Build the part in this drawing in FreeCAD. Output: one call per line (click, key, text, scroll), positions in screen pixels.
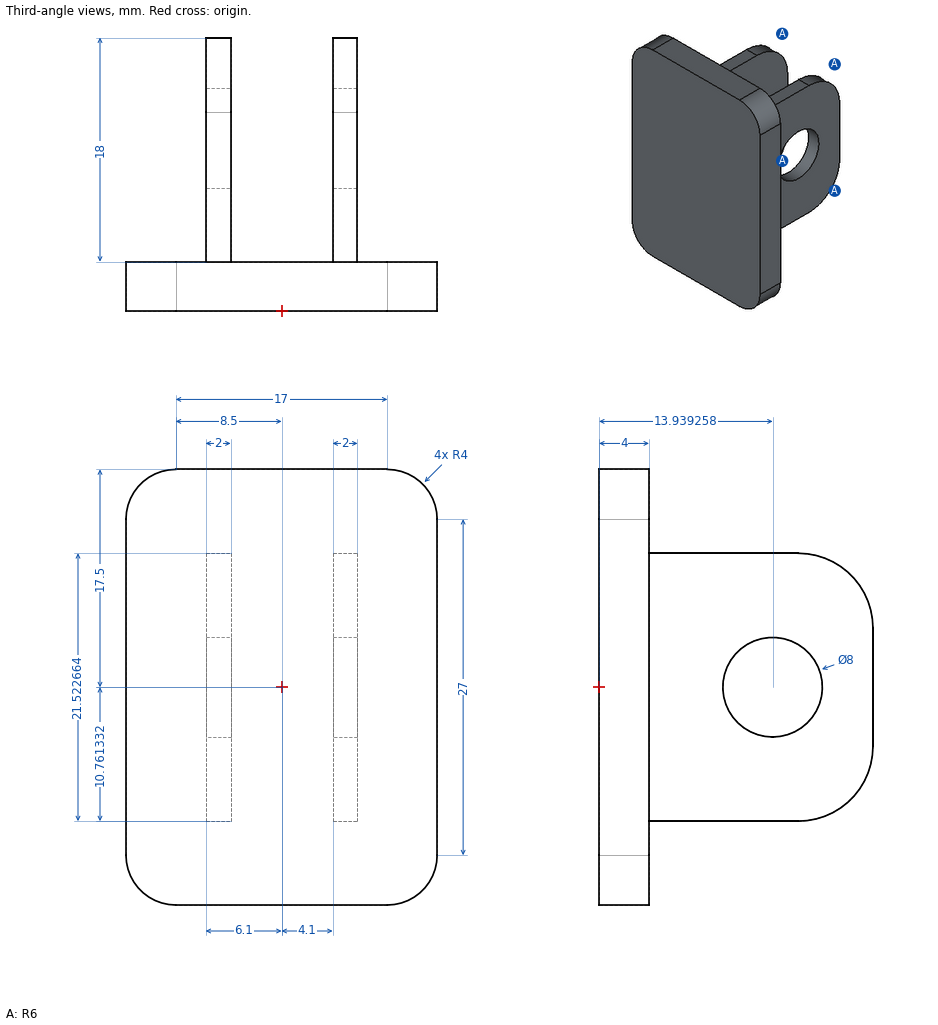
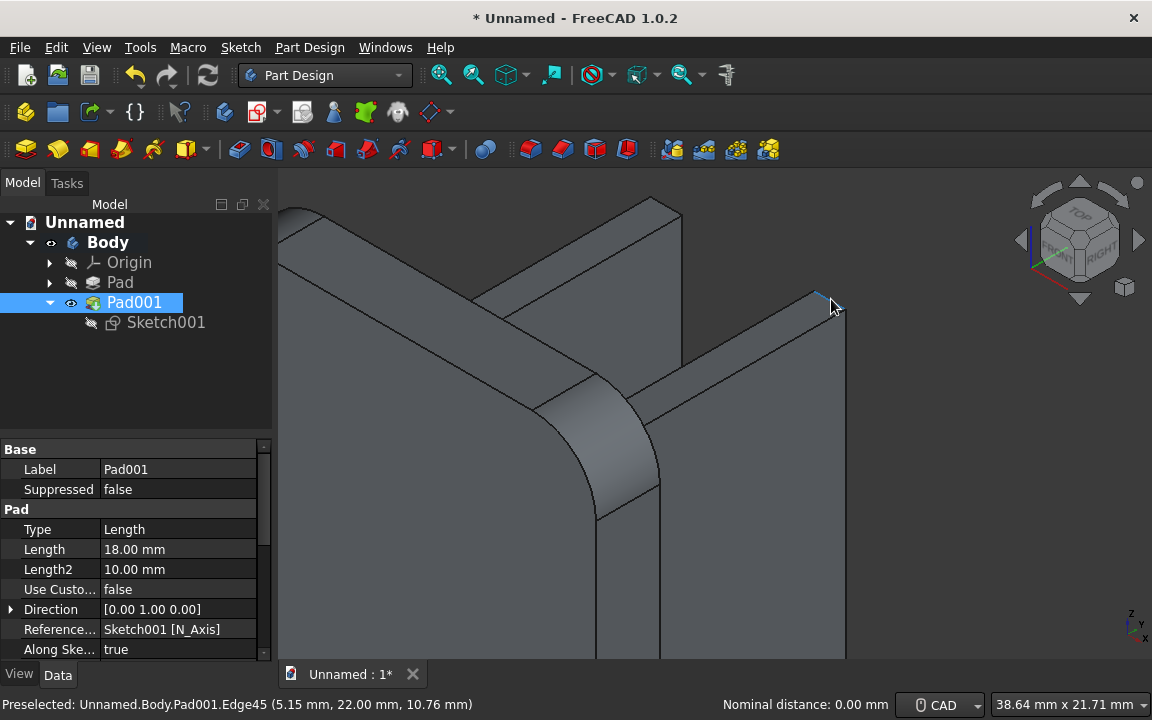
click(442, 76)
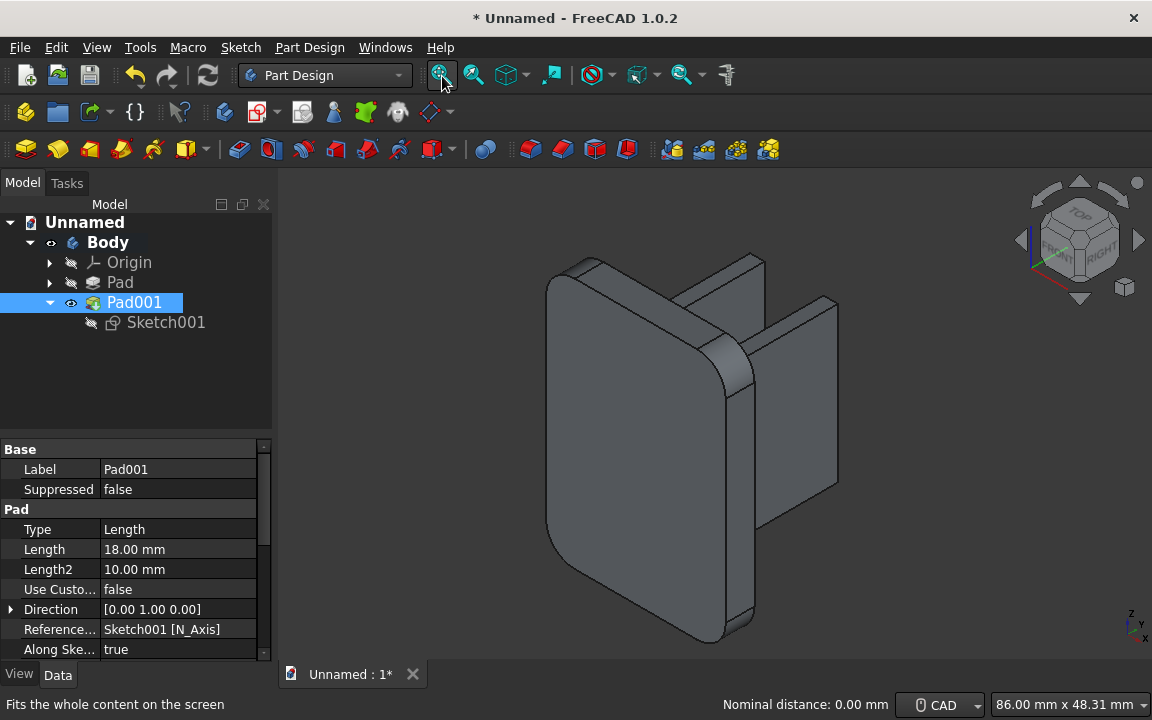
key(2)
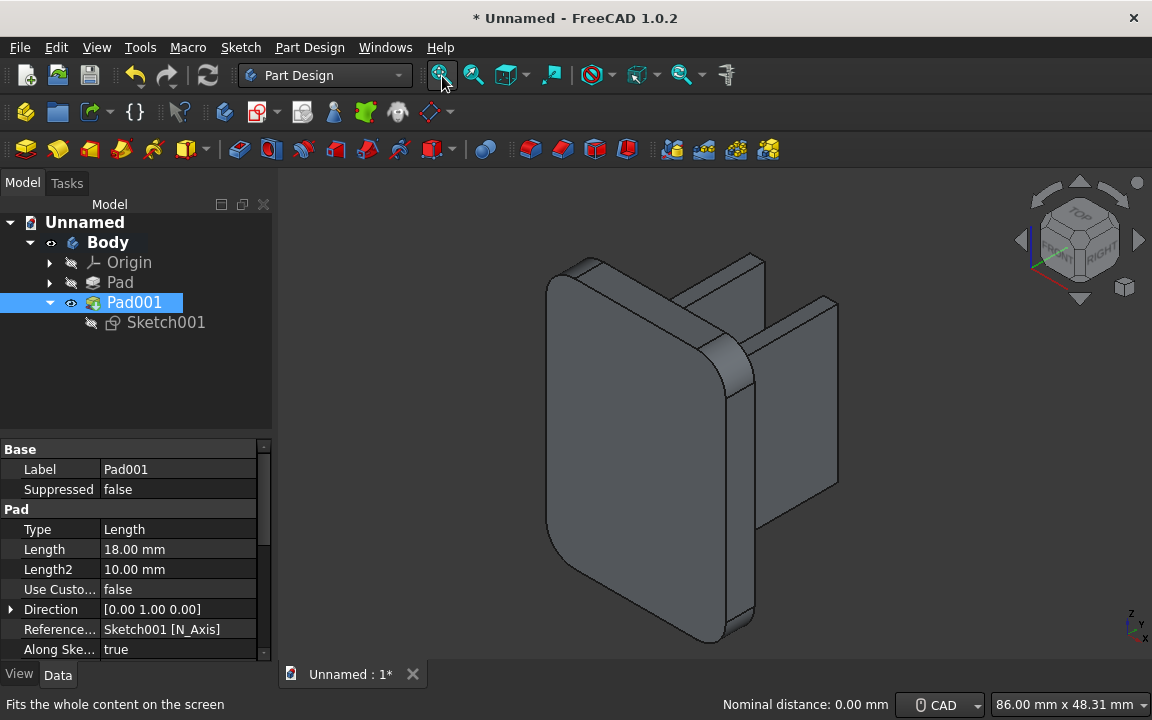
click(767, 301, ctrl)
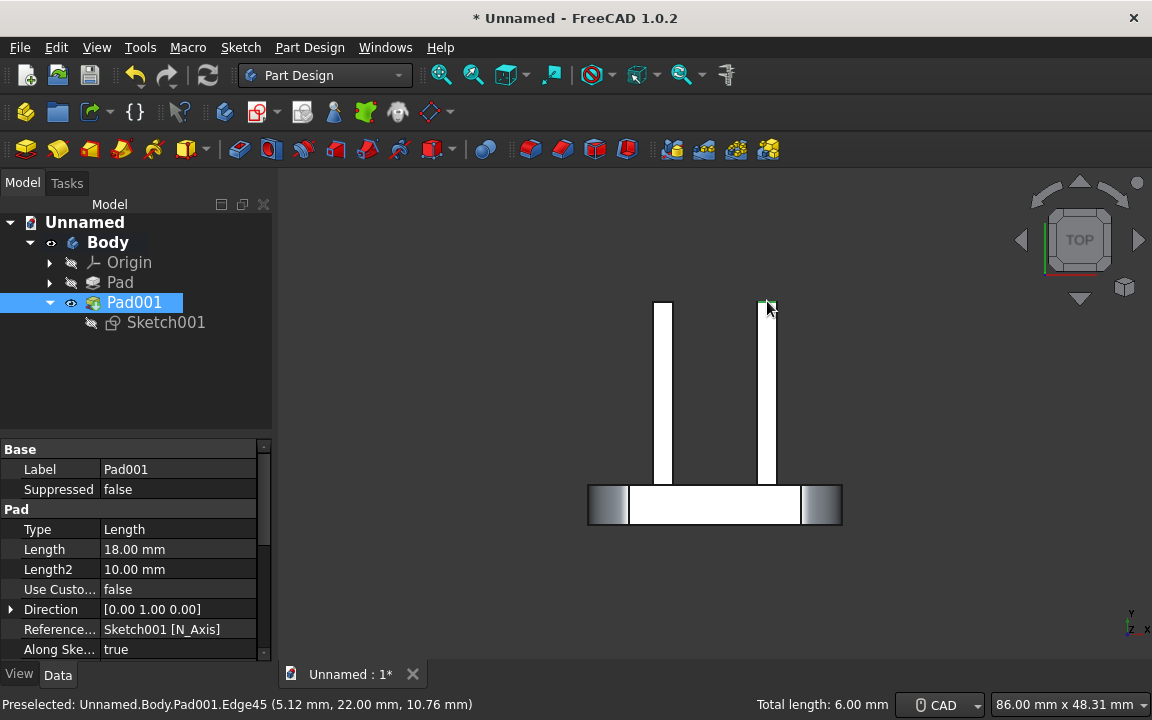
click(663, 301, ctrl)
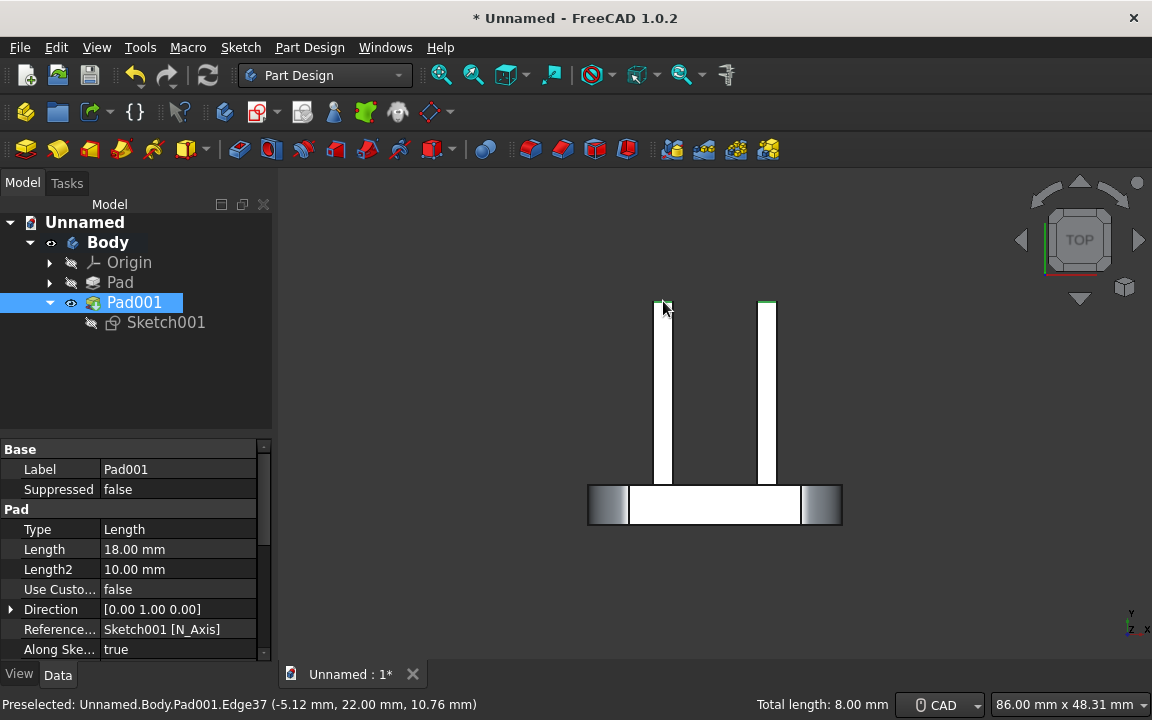
click(532, 150)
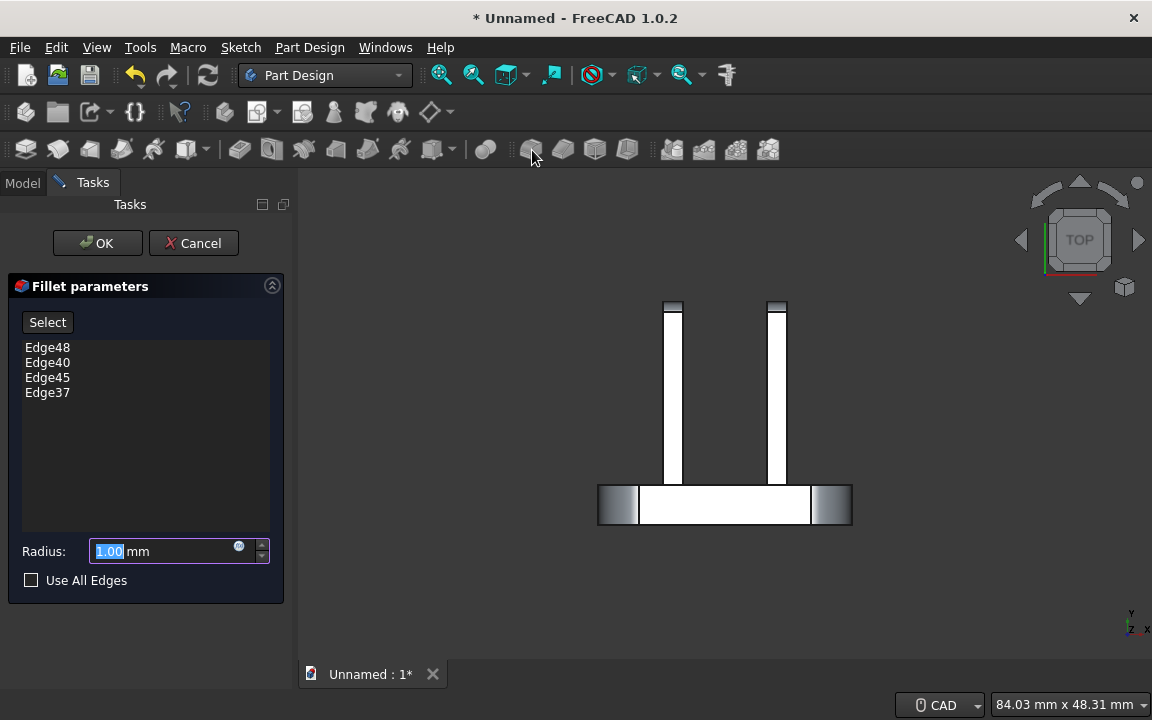
text(6)
key(Tab)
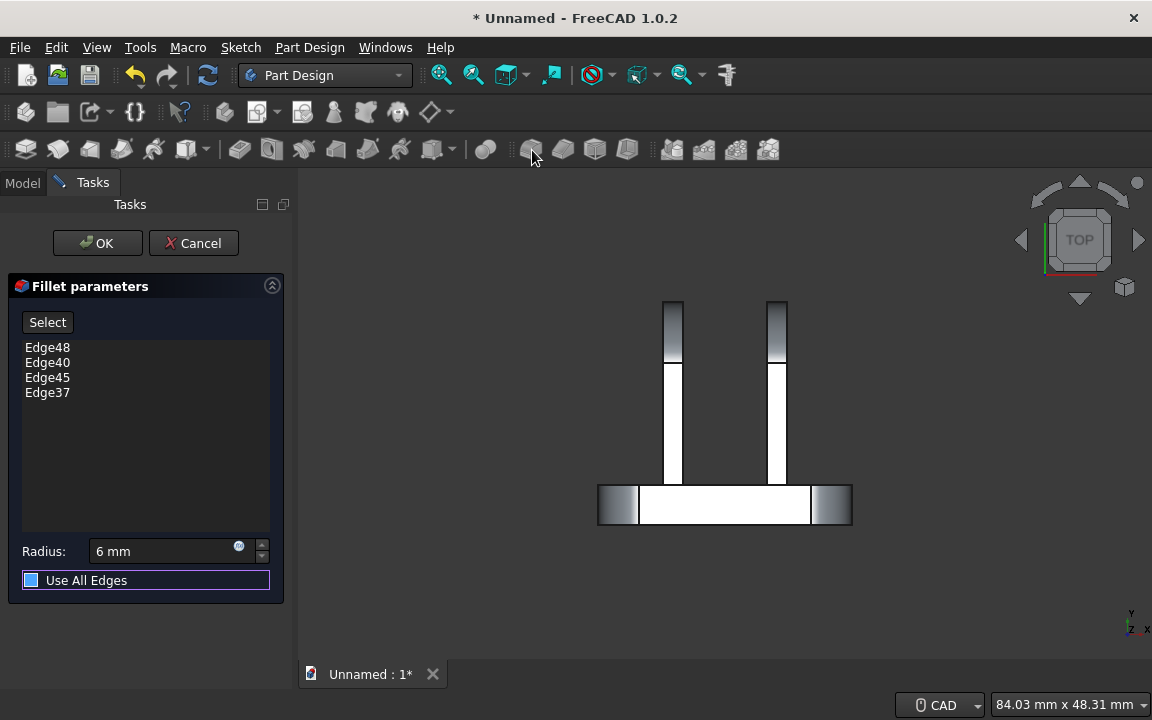
click(98, 243)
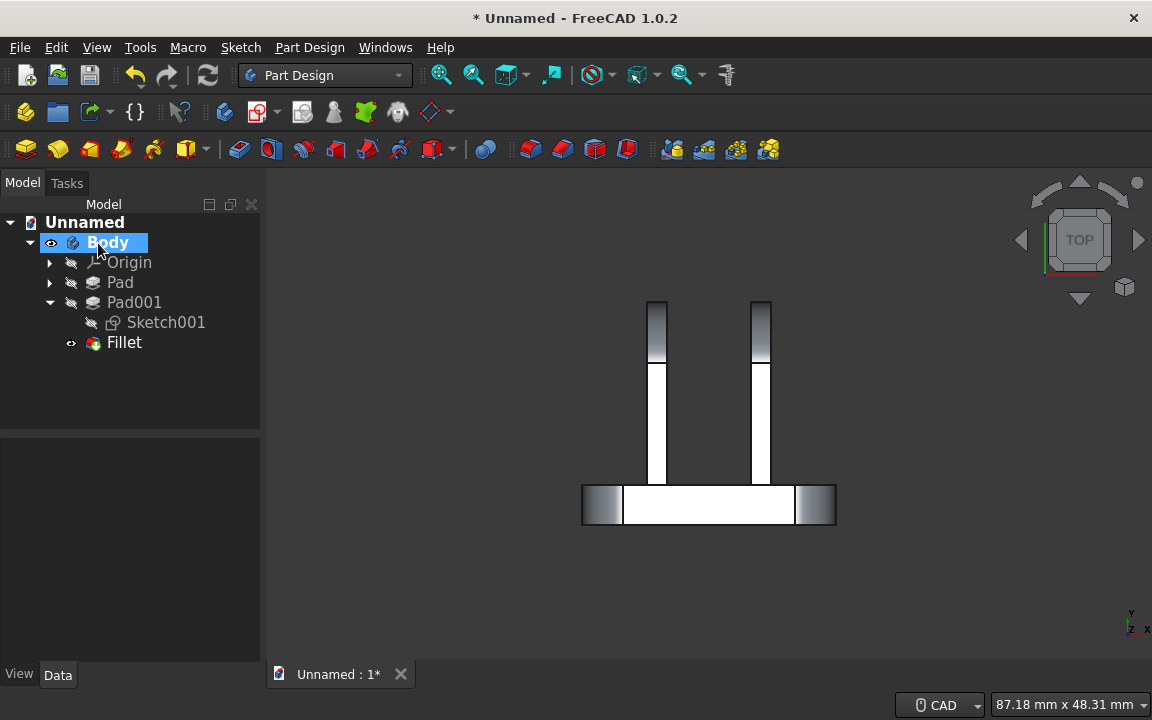
key(0)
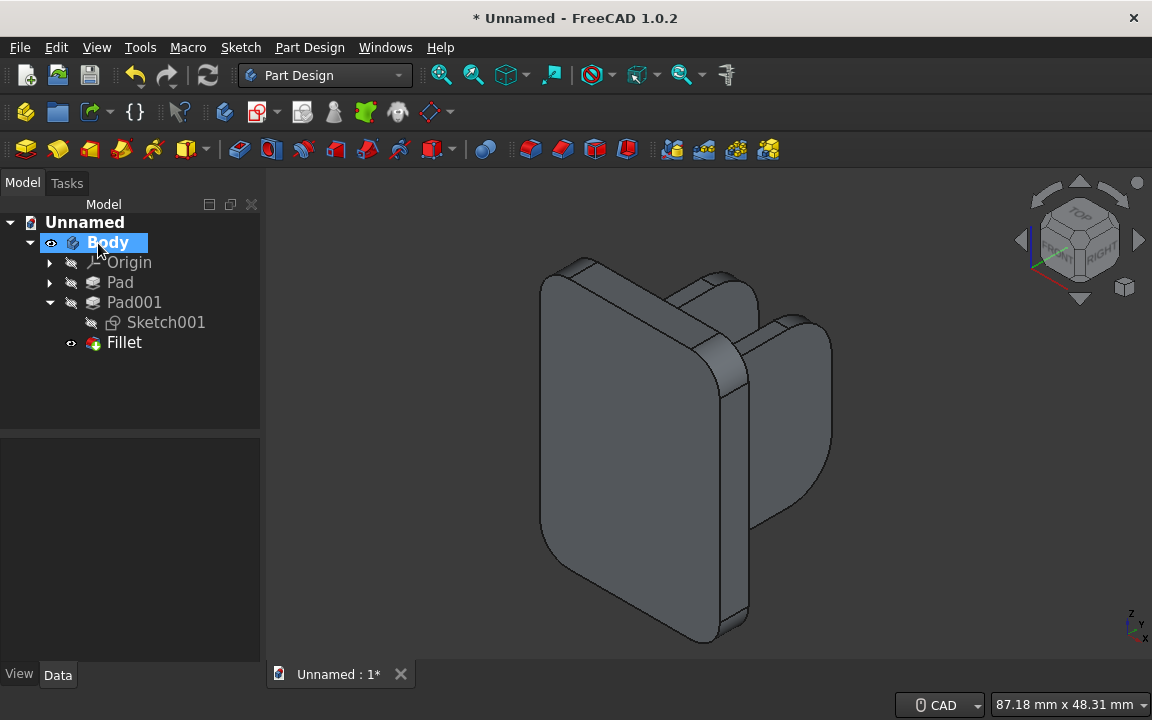
click(767, 430)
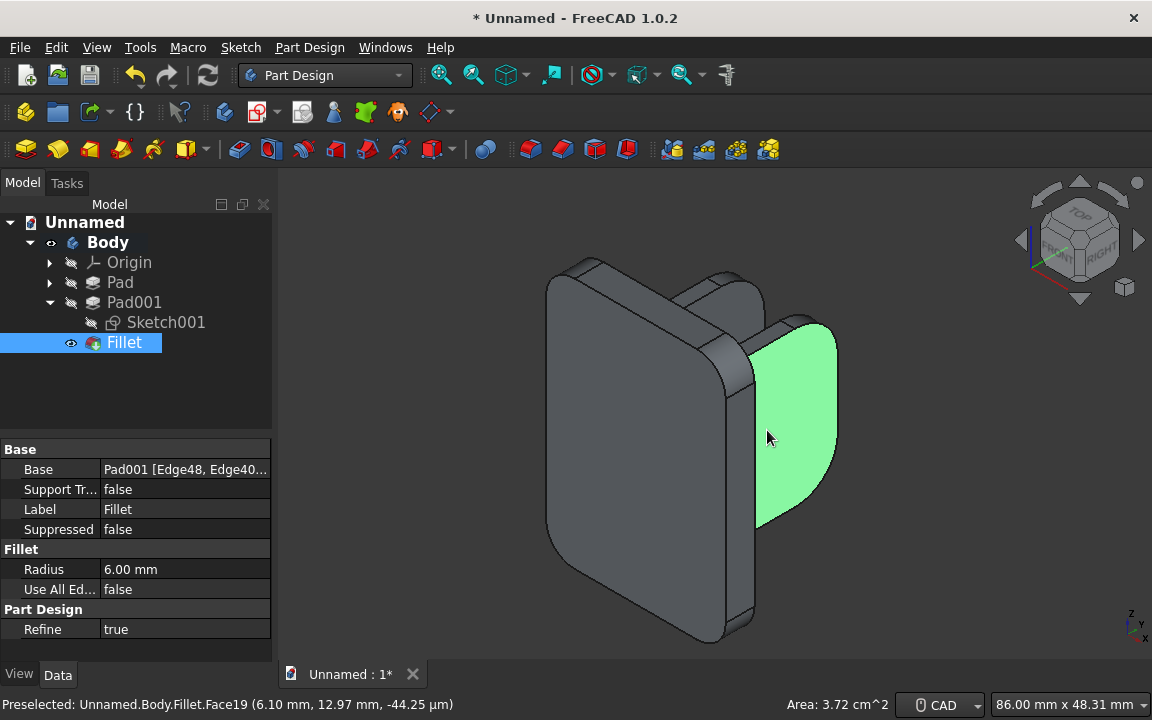
click(258, 112)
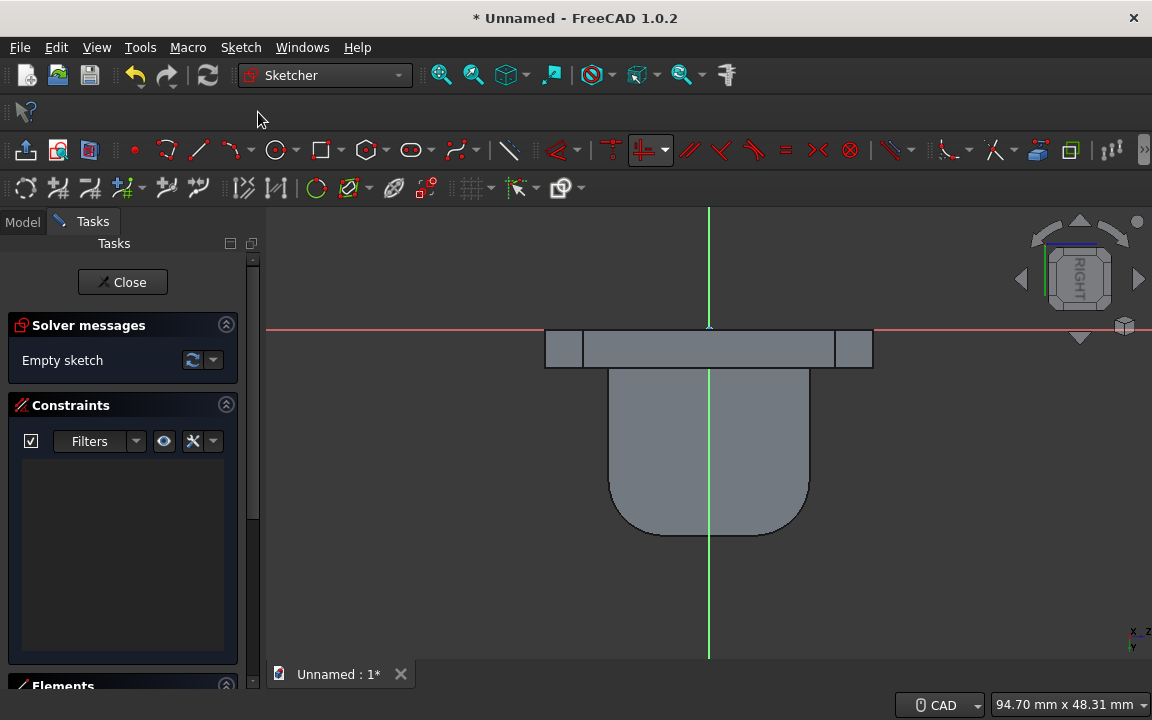
click(90, 150)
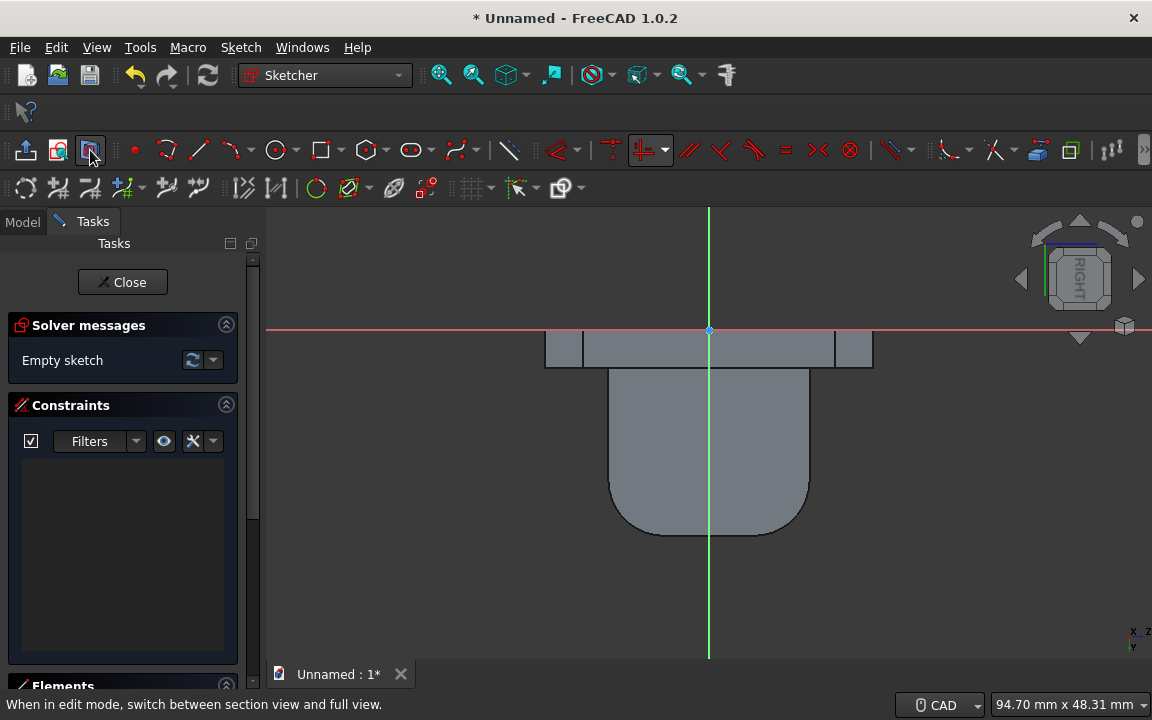
scroll(792, 391, up, 3)